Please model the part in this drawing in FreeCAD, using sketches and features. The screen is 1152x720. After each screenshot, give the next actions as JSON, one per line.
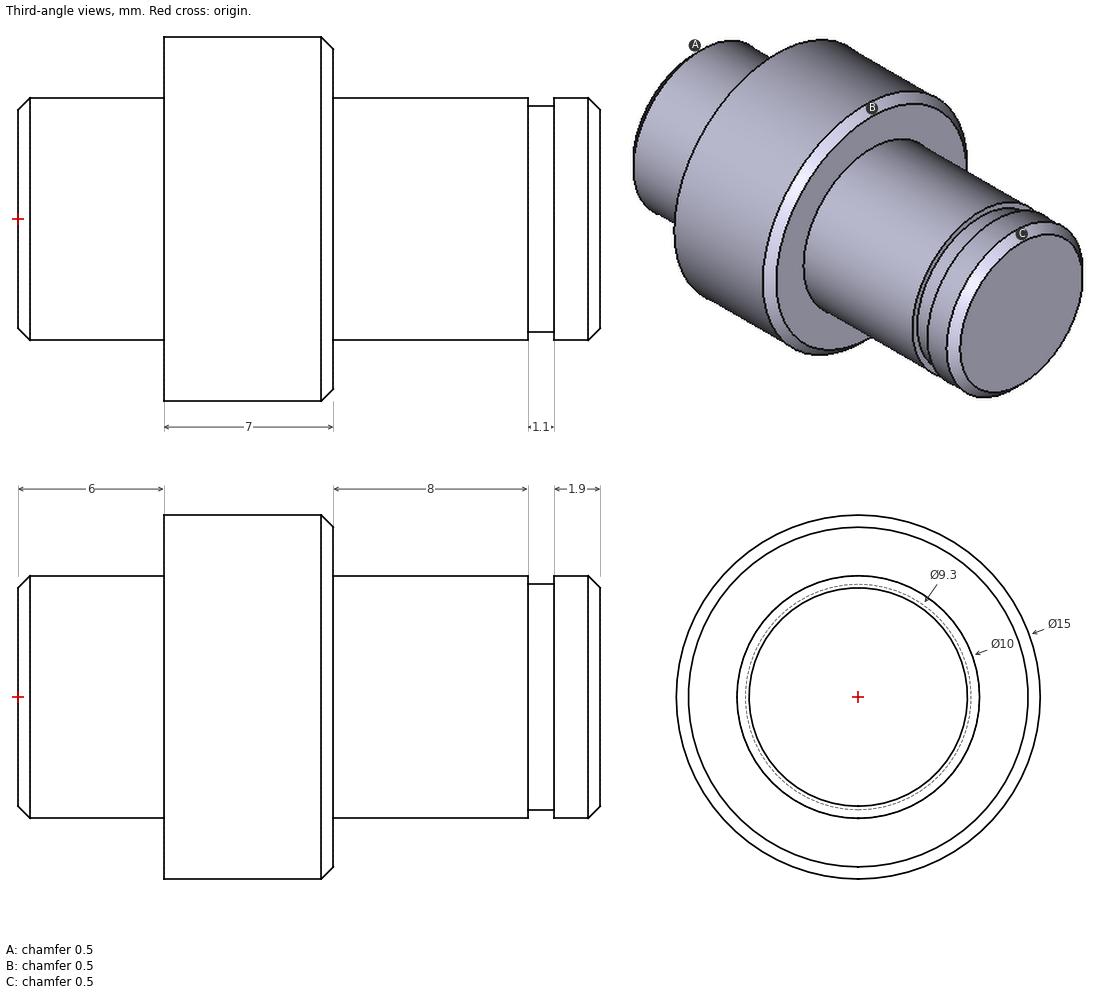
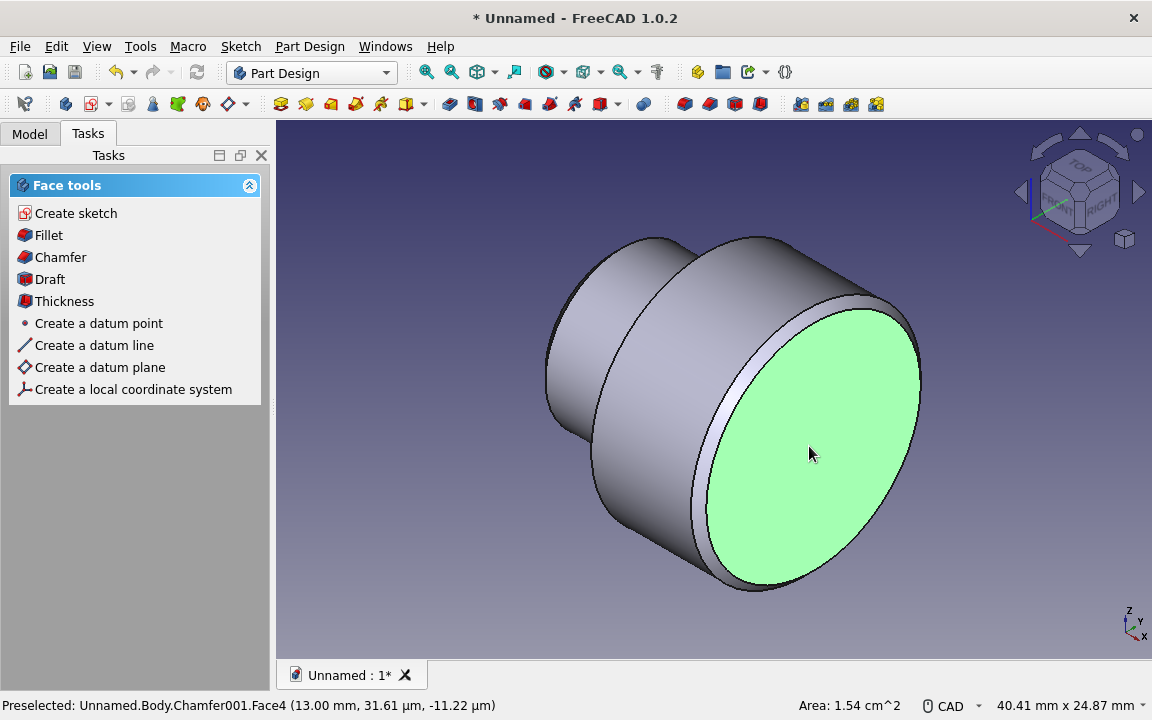
{"action": "left_click", "coordinate": [90, 104]}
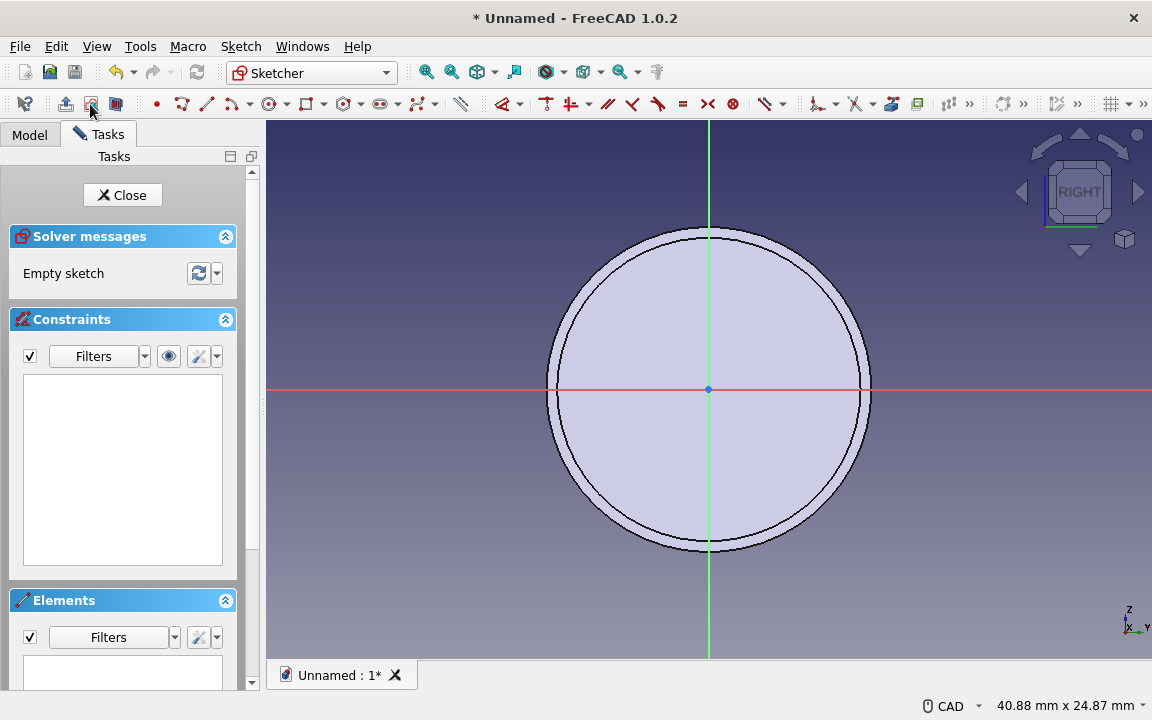
{"action": "scroll", "coordinate": [848, 389], "scroll_direction": "up", "scroll_amount": 2}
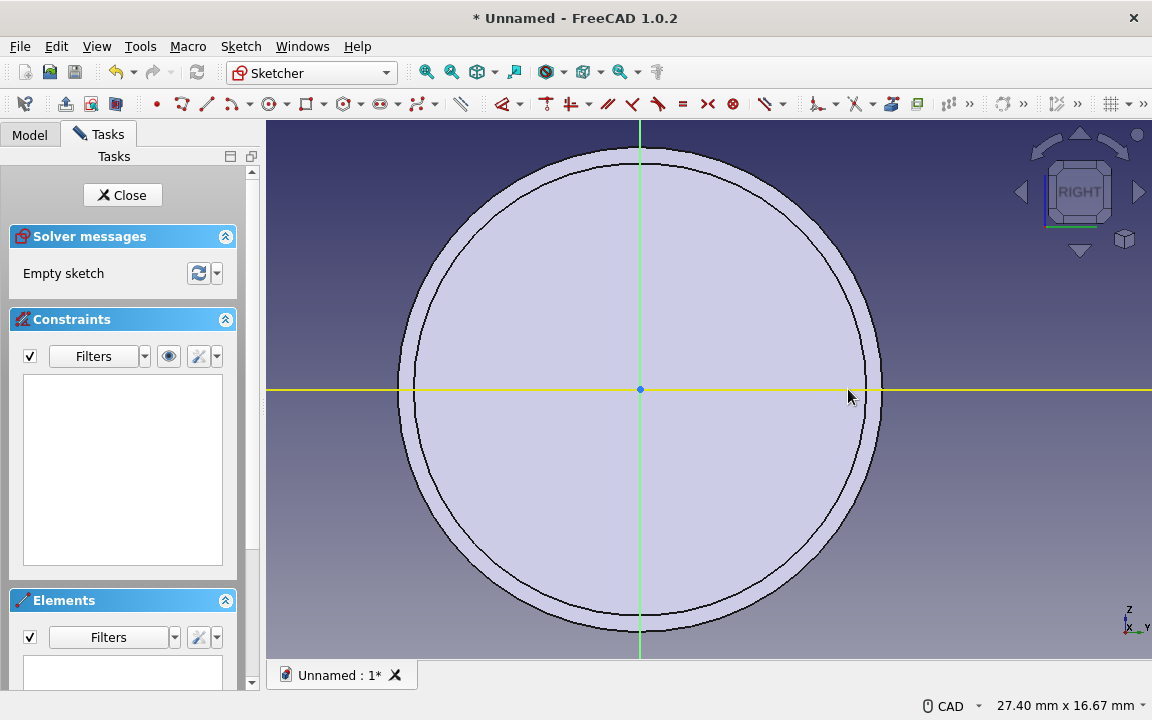
{"action": "key", "text": "g c"}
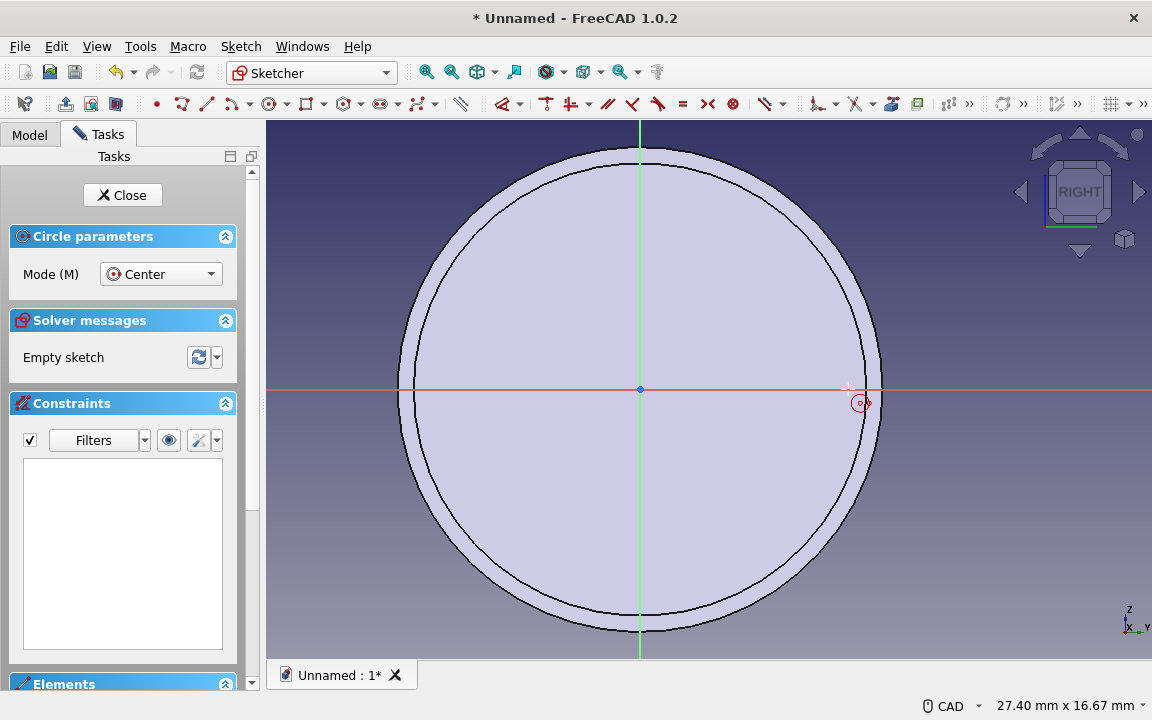
{"action": "left_click", "coordinate": [640, 389]}
{"action": "mouse_move", "coordinate": [754, 275]}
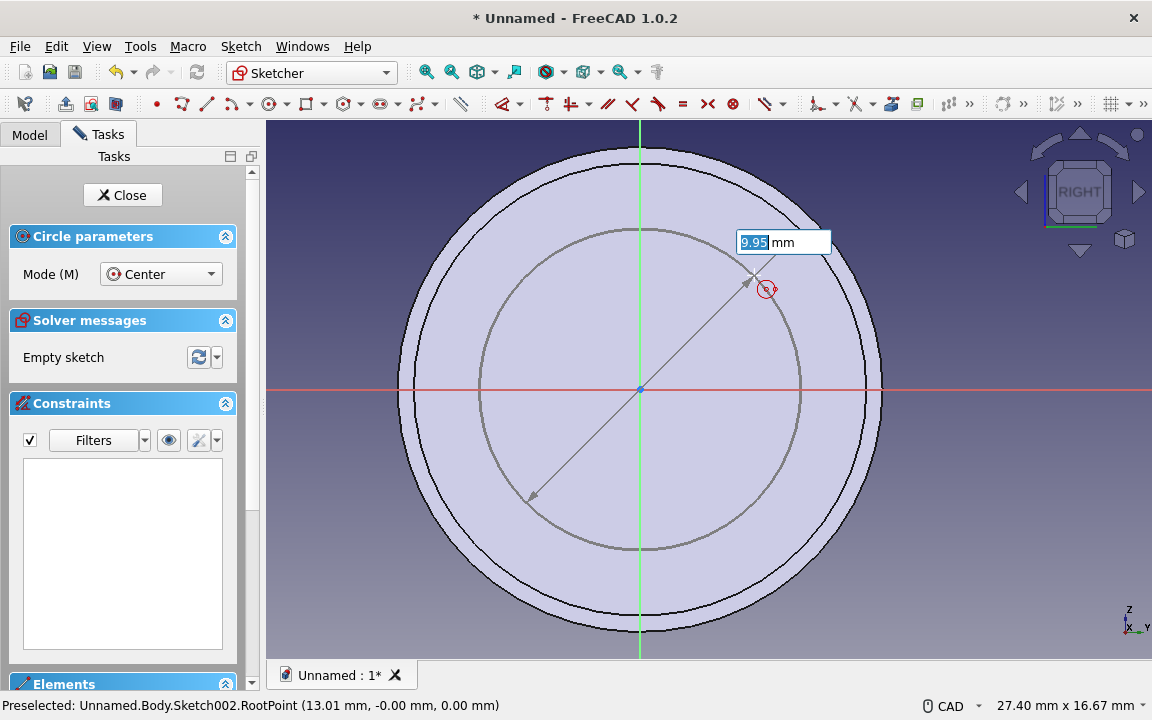
{"action": "type", "text": "10"}
{"action": "key", "text": "Return"}
{"action": "key", "text": "Escape"}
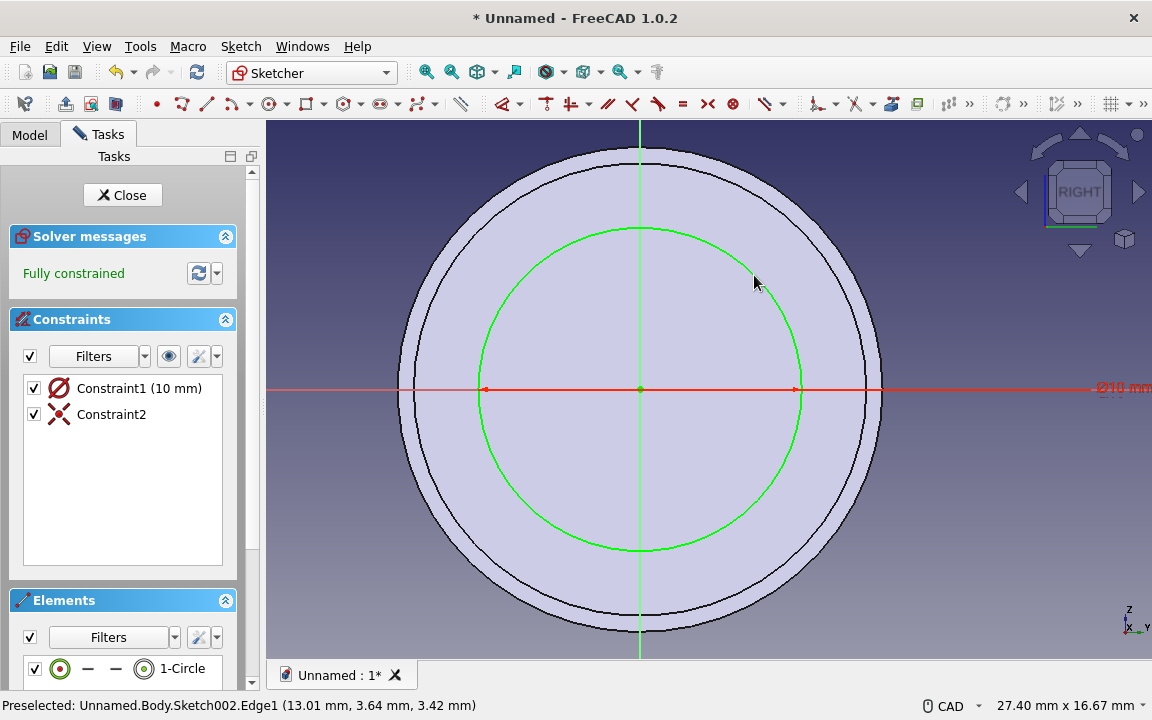
{"action": "left_click", "coordinate": [123, 195]}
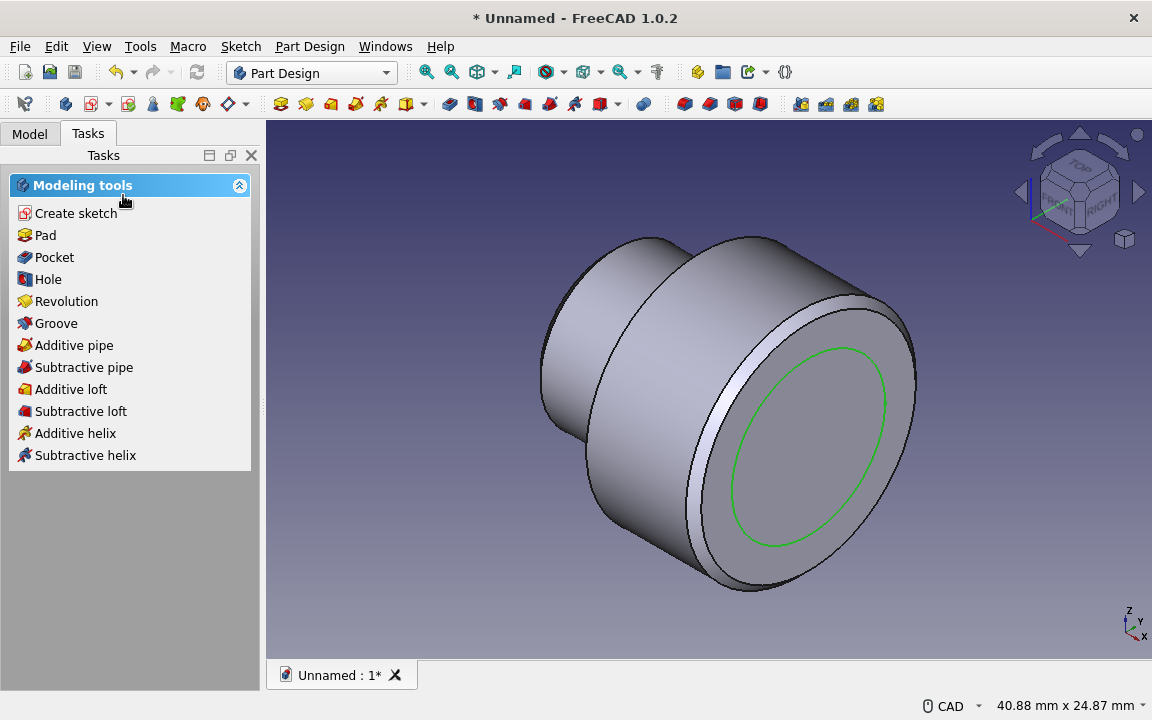
{"action": "left_click", "coordinate": [281, 104]}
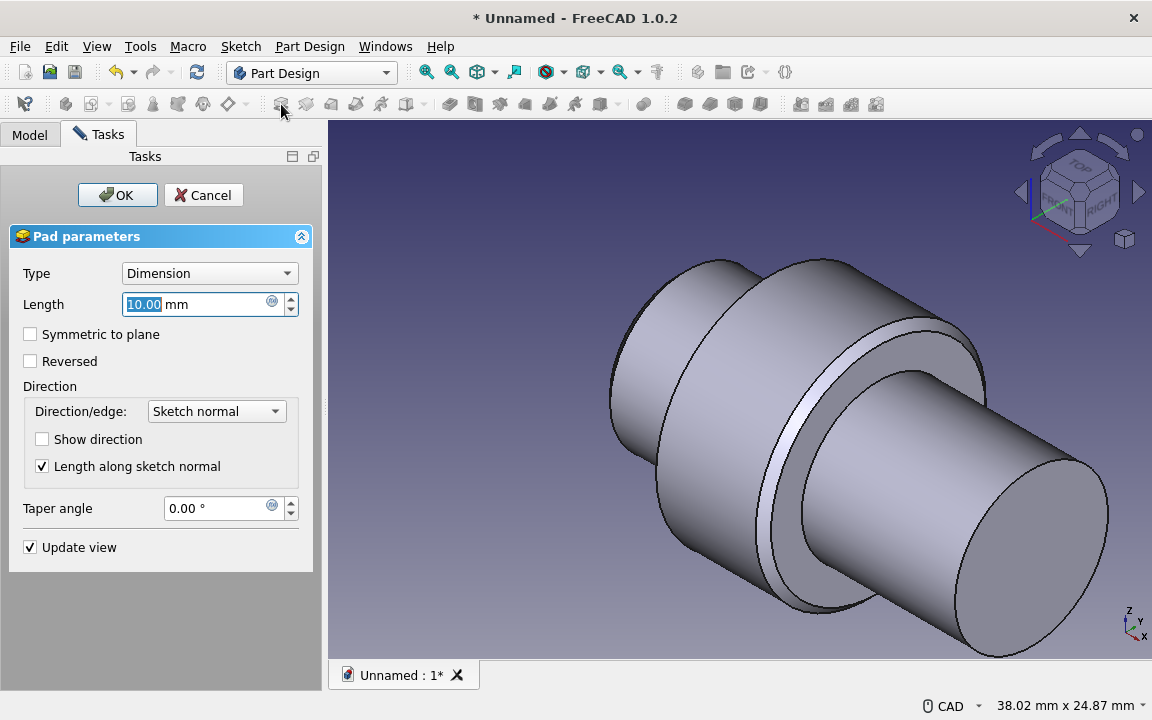
{"action": "type", "text": "8"}
{"action": "key", "text": "Tab"}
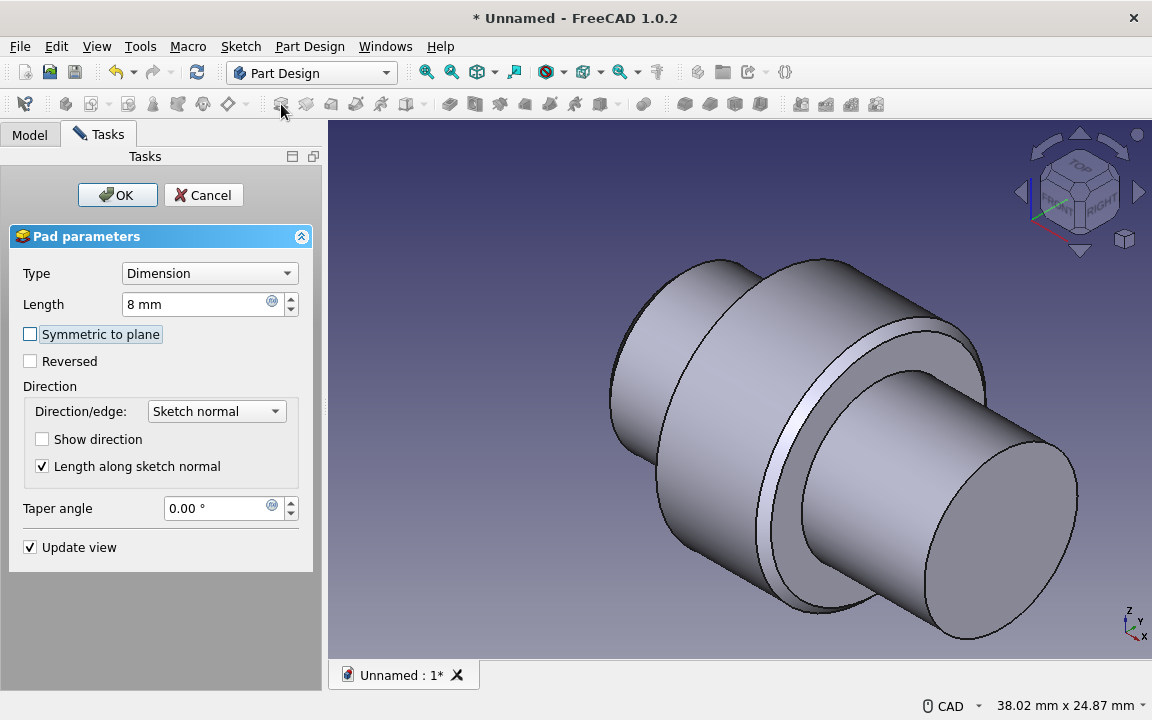
{"action": "left_click", "coordinate": [118, 195]}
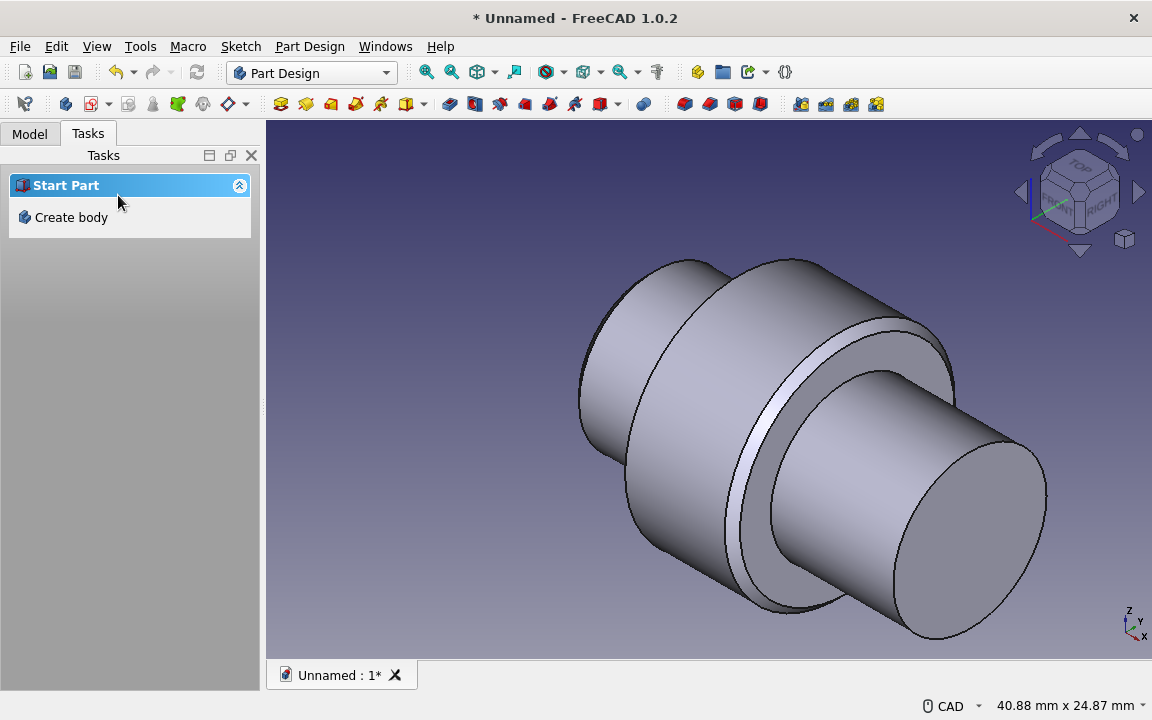
{"action": "key", "text": "v f"}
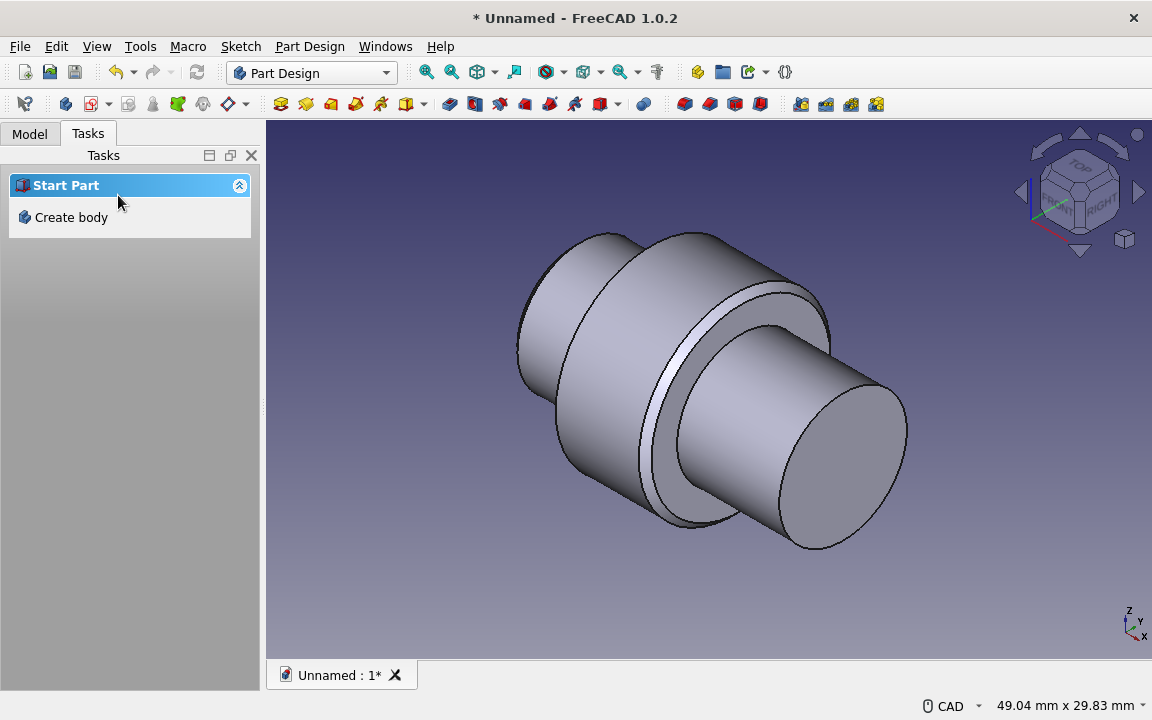
{"action": "left_click", "coordinate": [843, 466]}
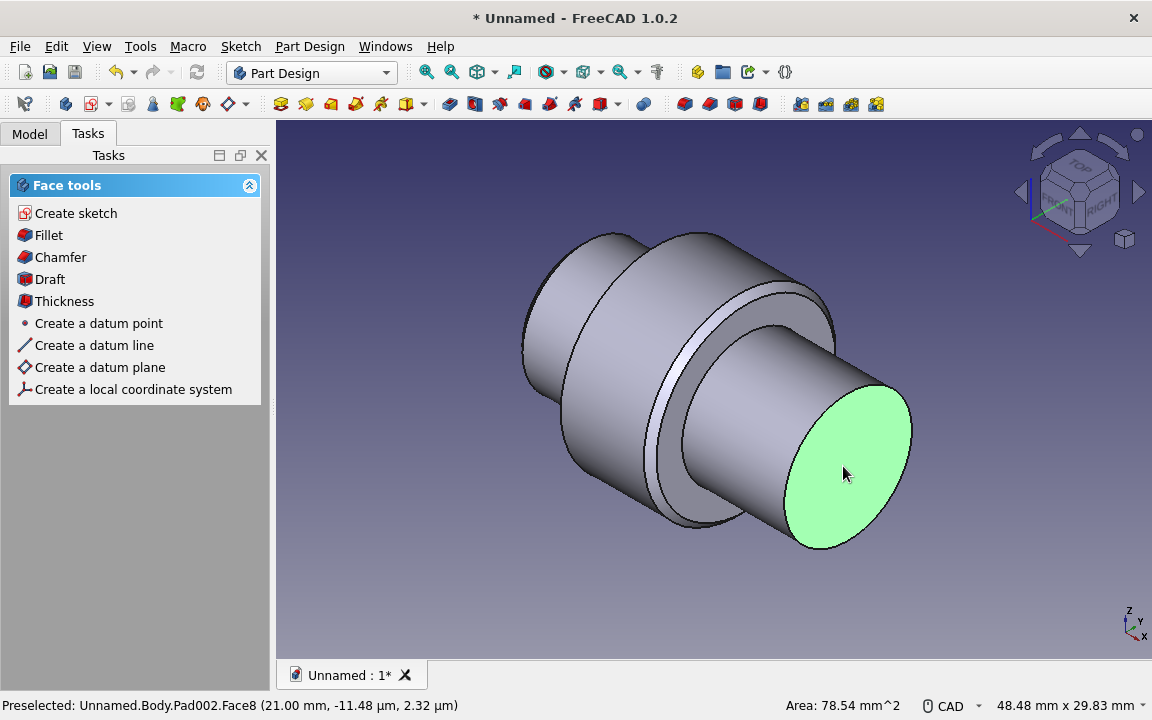
{"action": "left_click", "coordinate": [90, 104]}